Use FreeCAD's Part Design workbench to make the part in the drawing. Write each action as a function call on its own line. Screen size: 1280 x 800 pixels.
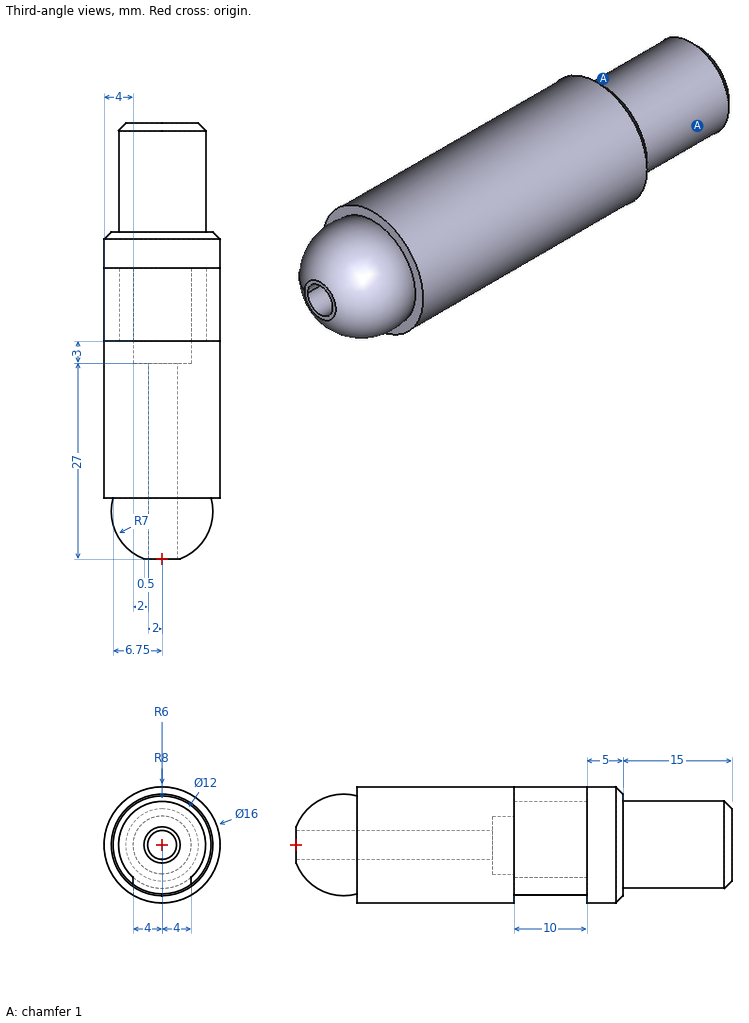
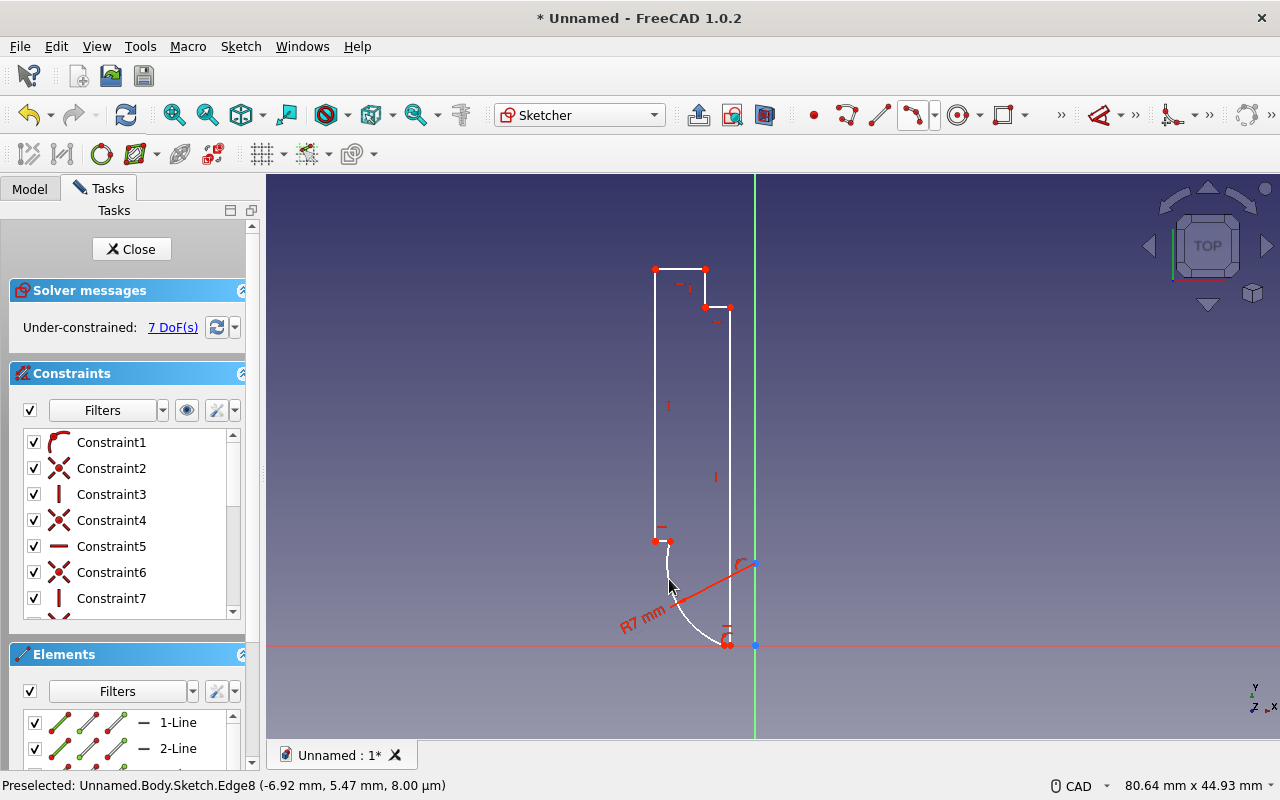
scroll(720, 307, up, 3)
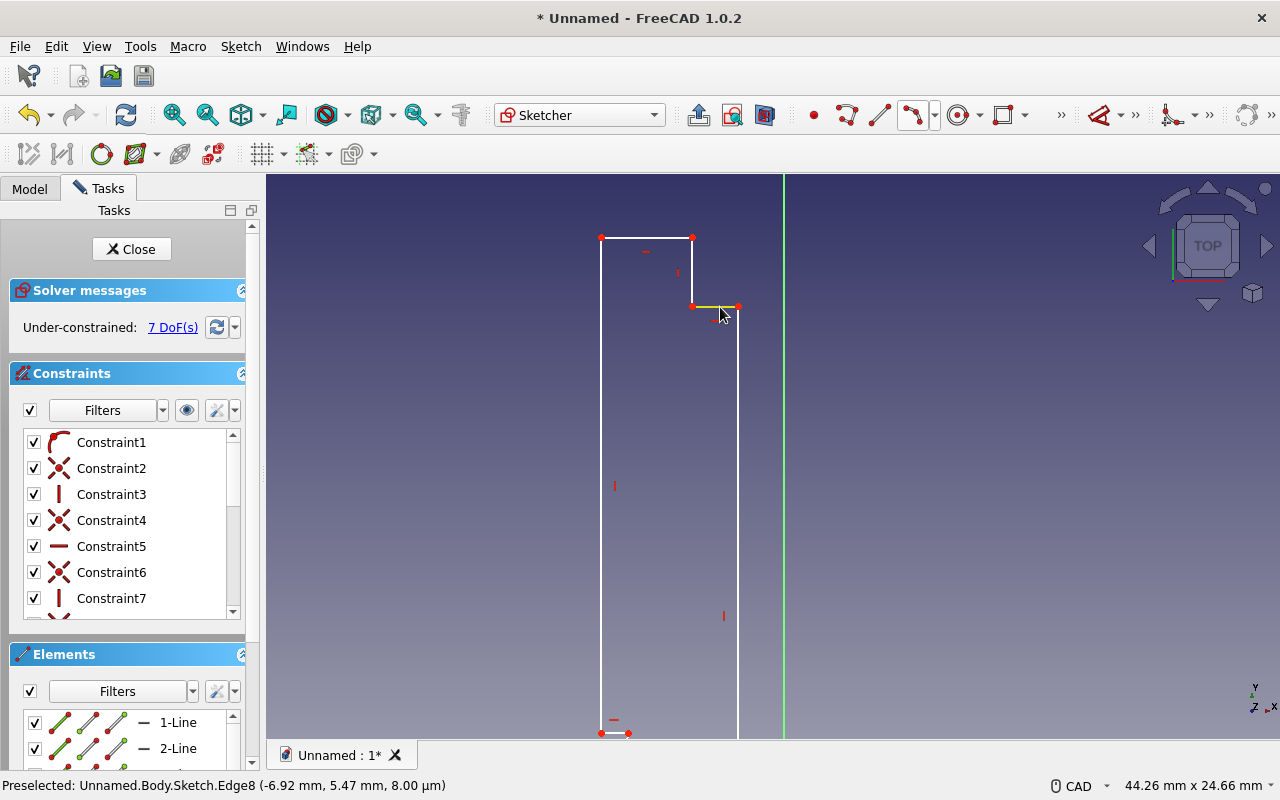
click(720, 307)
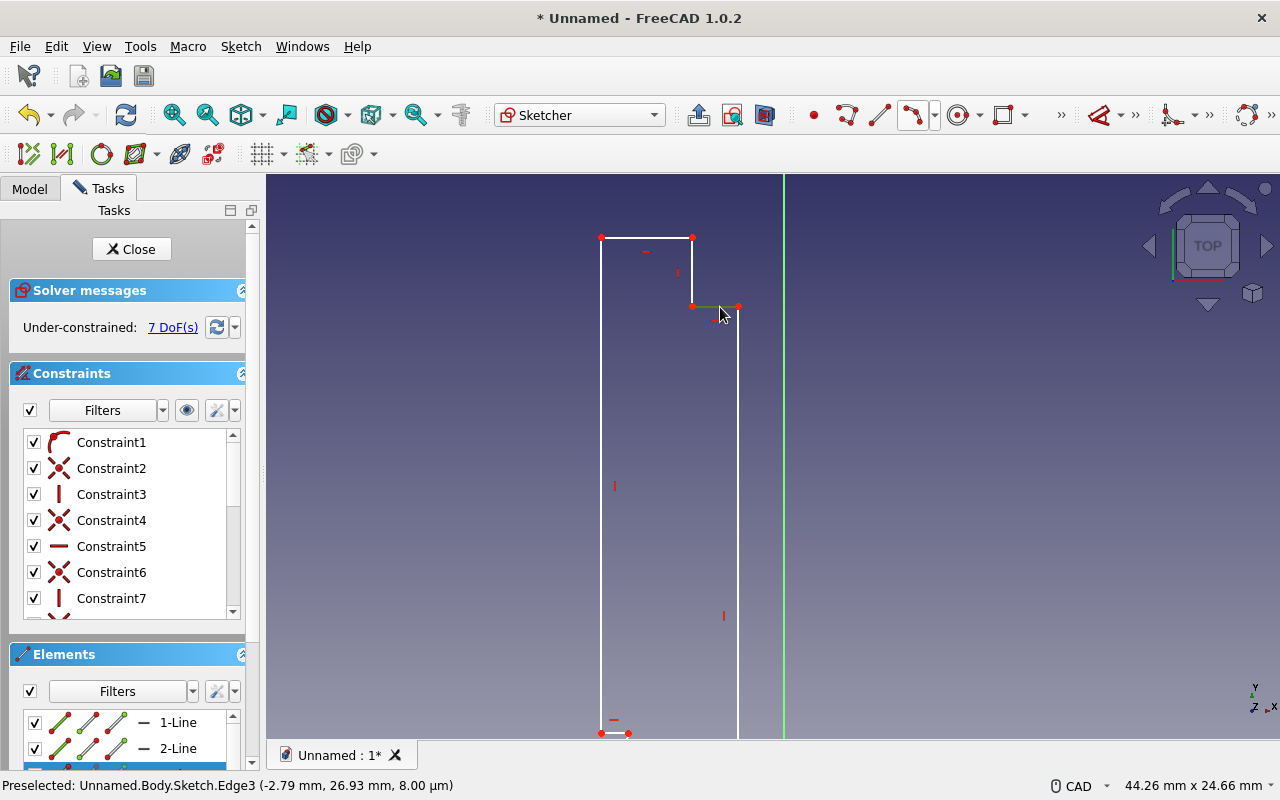
key(l)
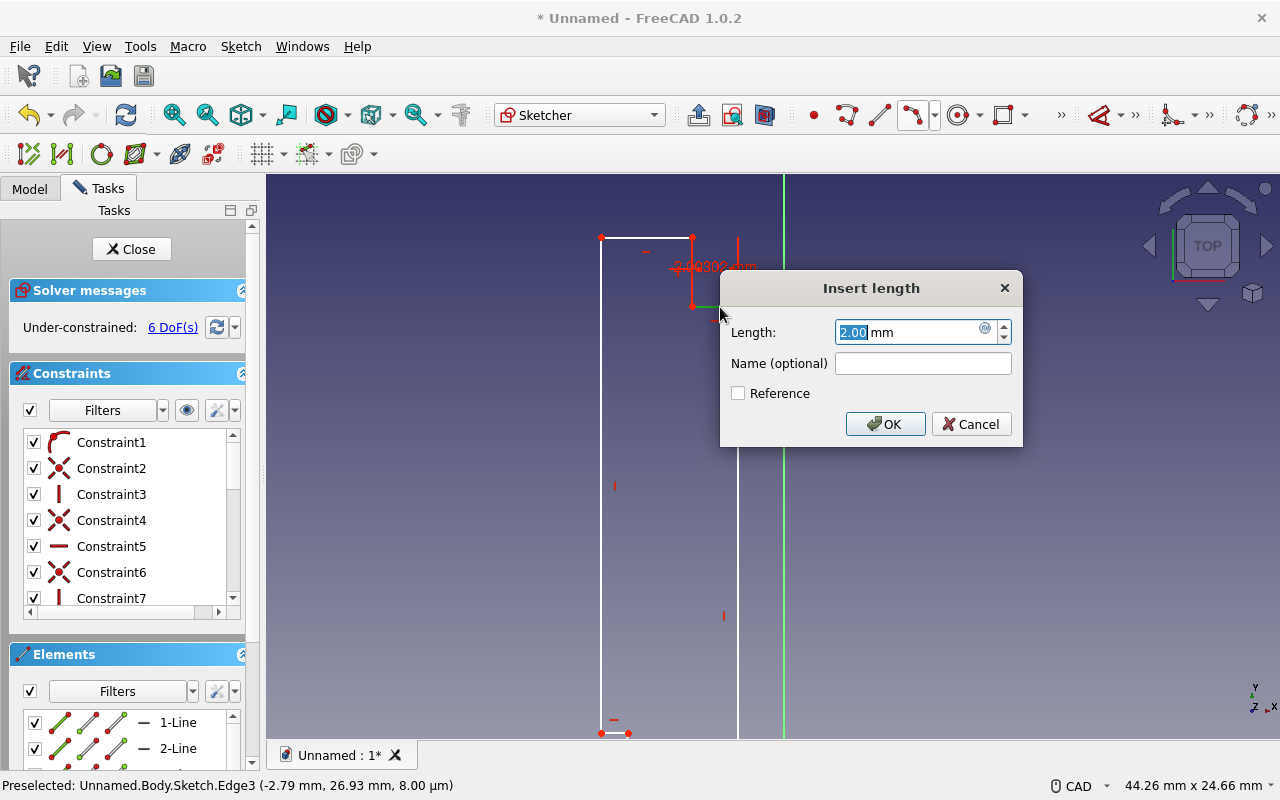
text(2)
key(Return)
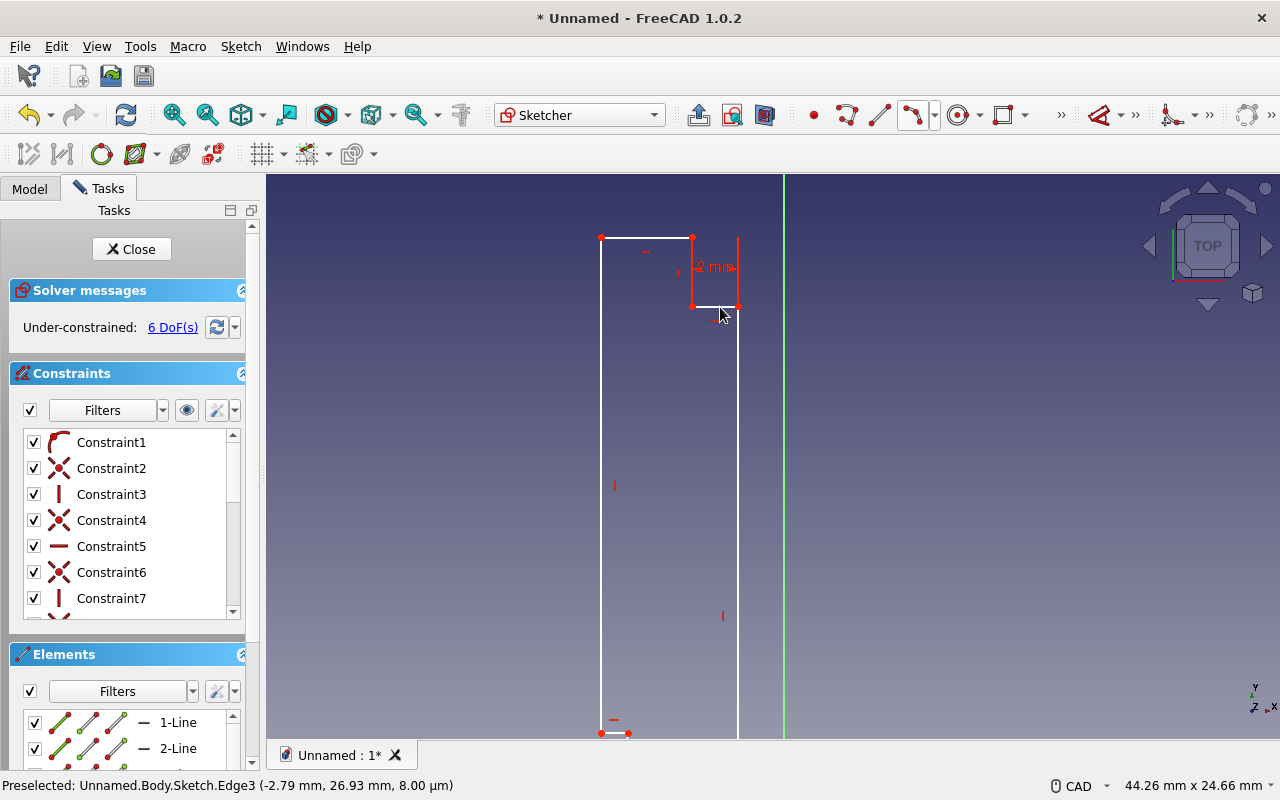
click(692, 286)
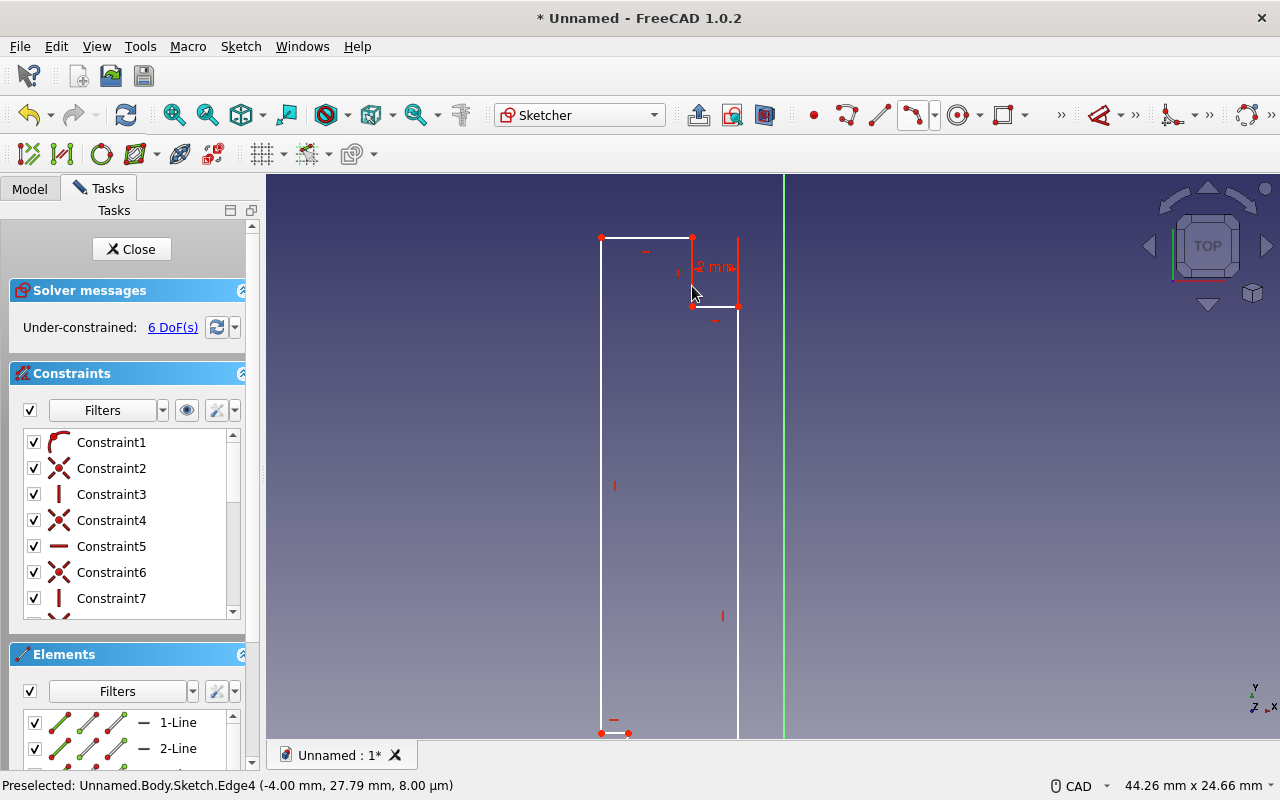
key(i)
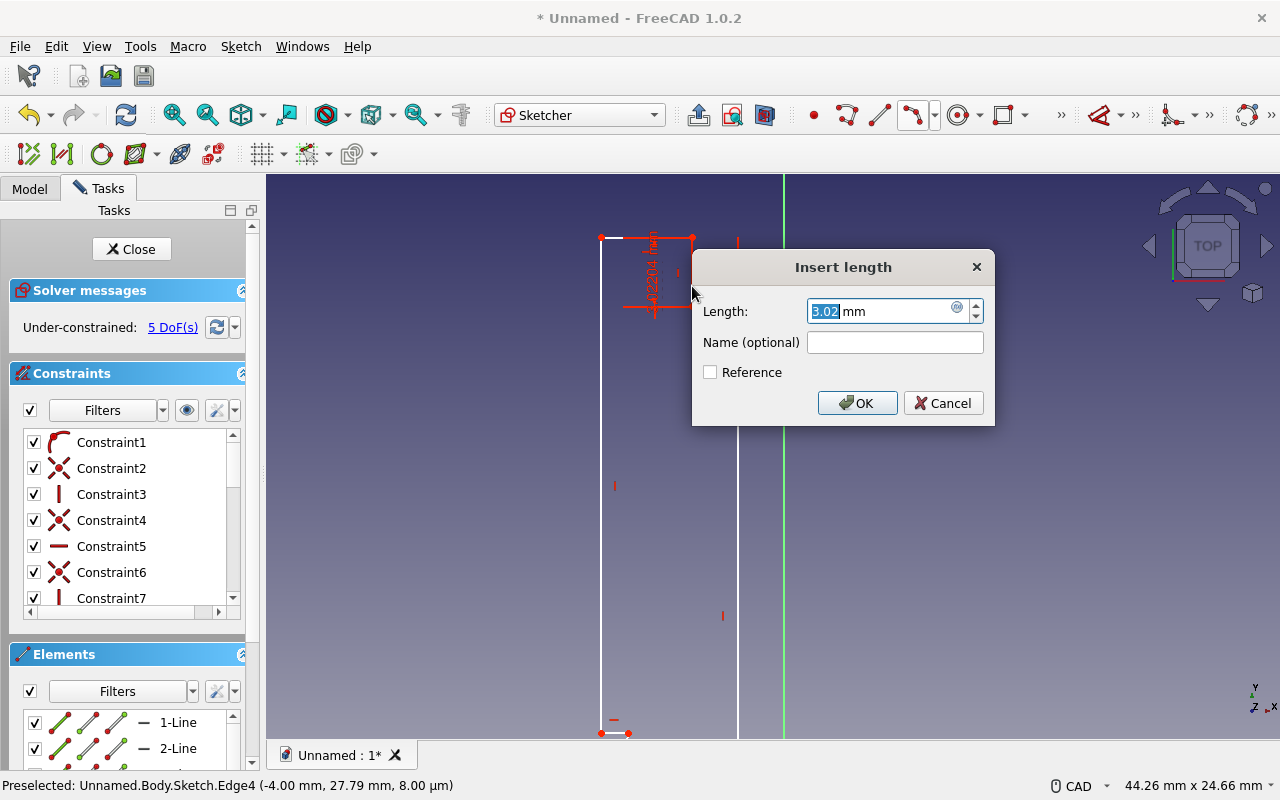
text(3)
key(Return)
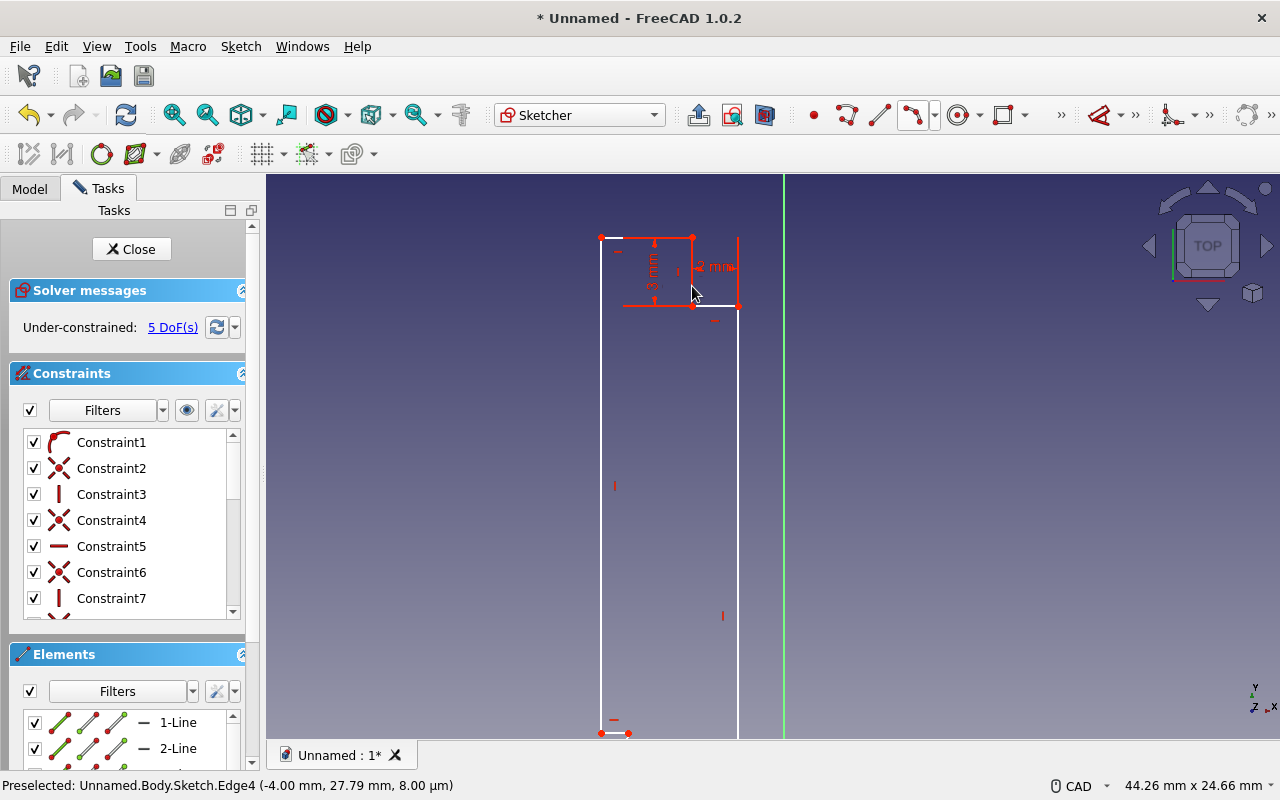
click(665, 238)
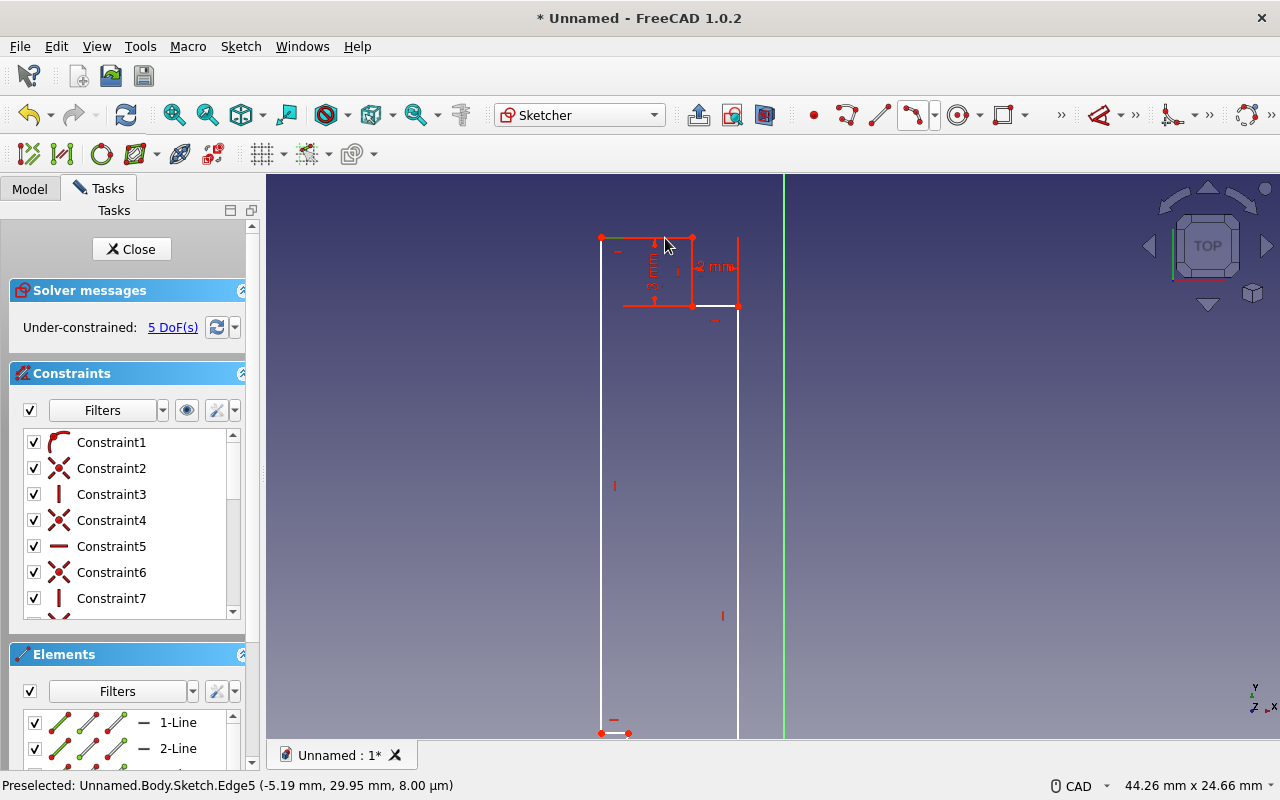
key(l)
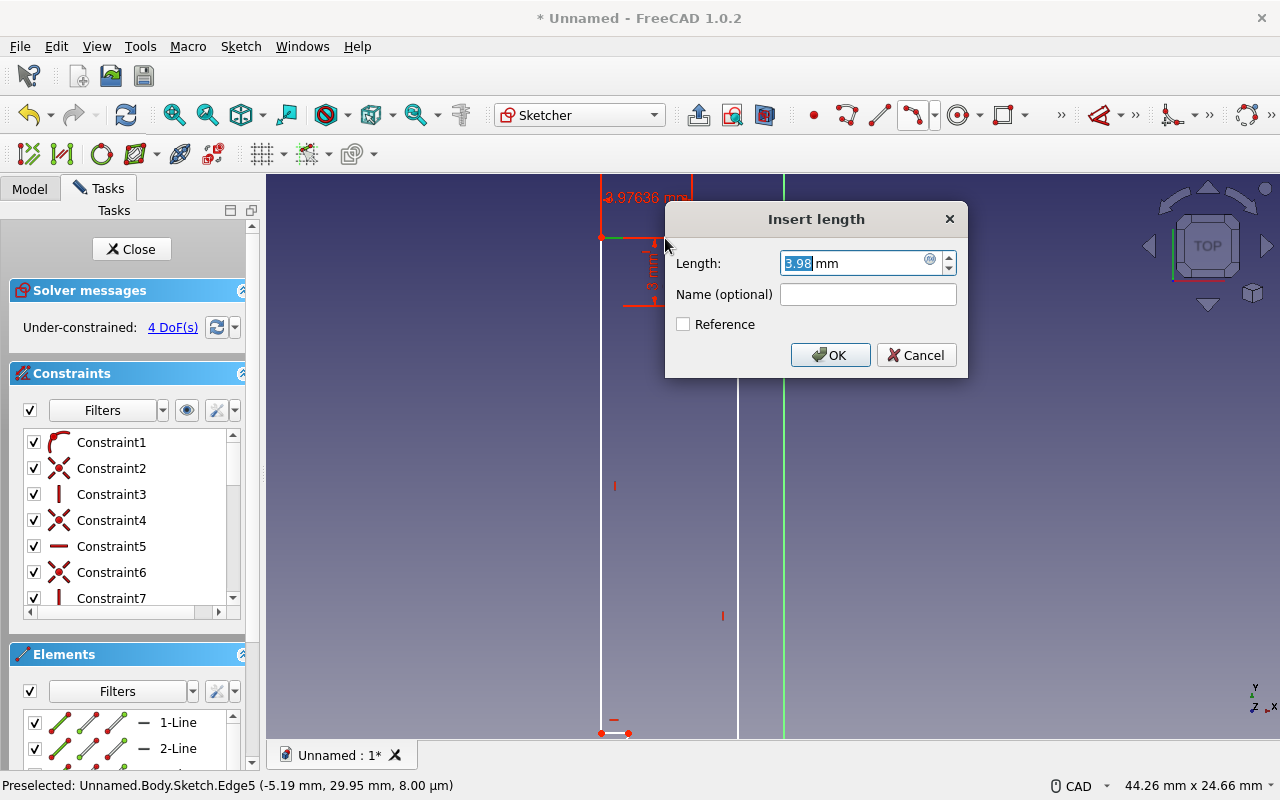
text(4)
key(Return)